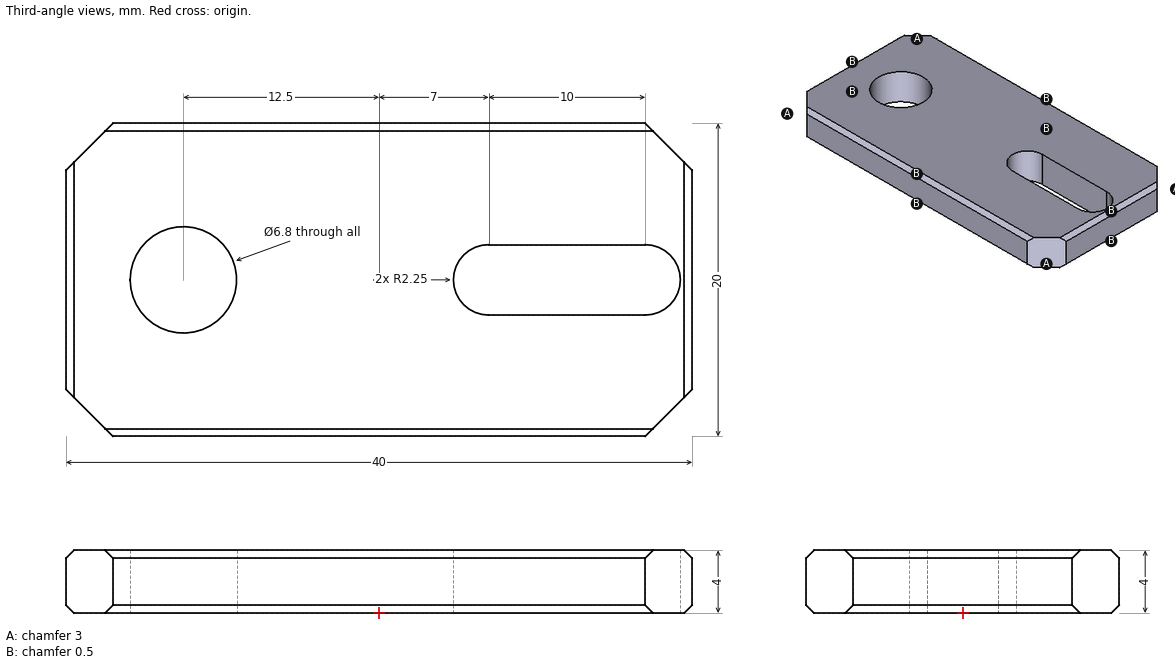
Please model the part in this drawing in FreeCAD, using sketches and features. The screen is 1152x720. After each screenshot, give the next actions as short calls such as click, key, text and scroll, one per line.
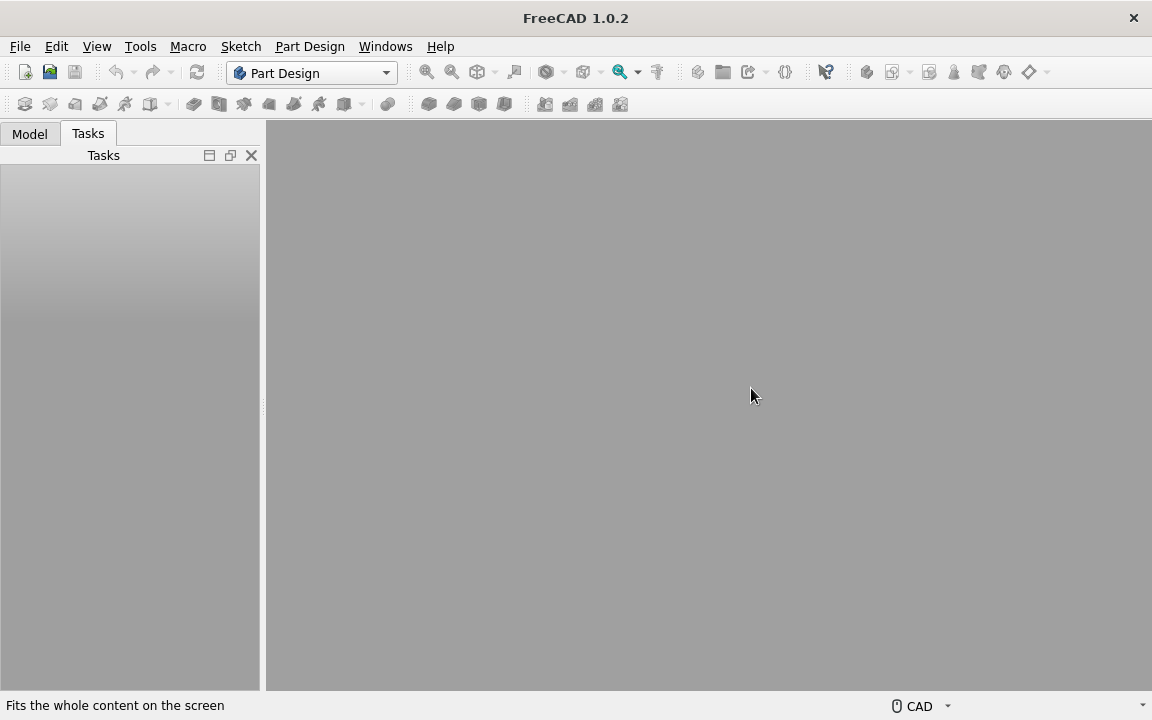
click(25, 72)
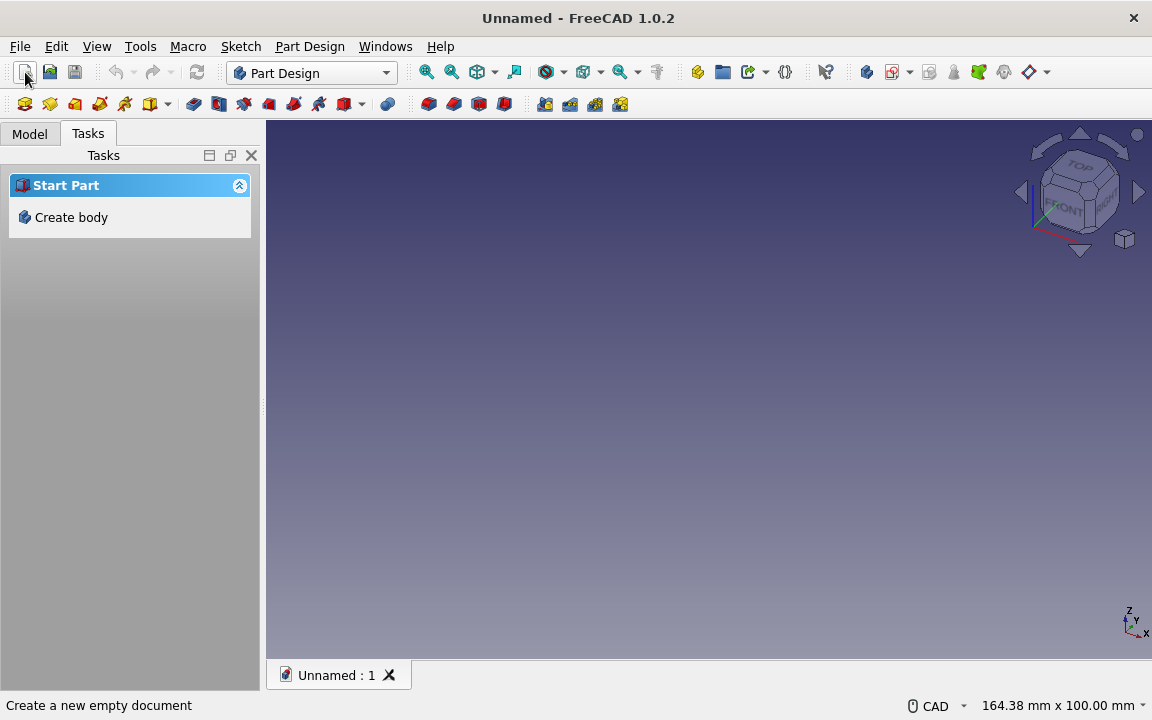
click(892, 72)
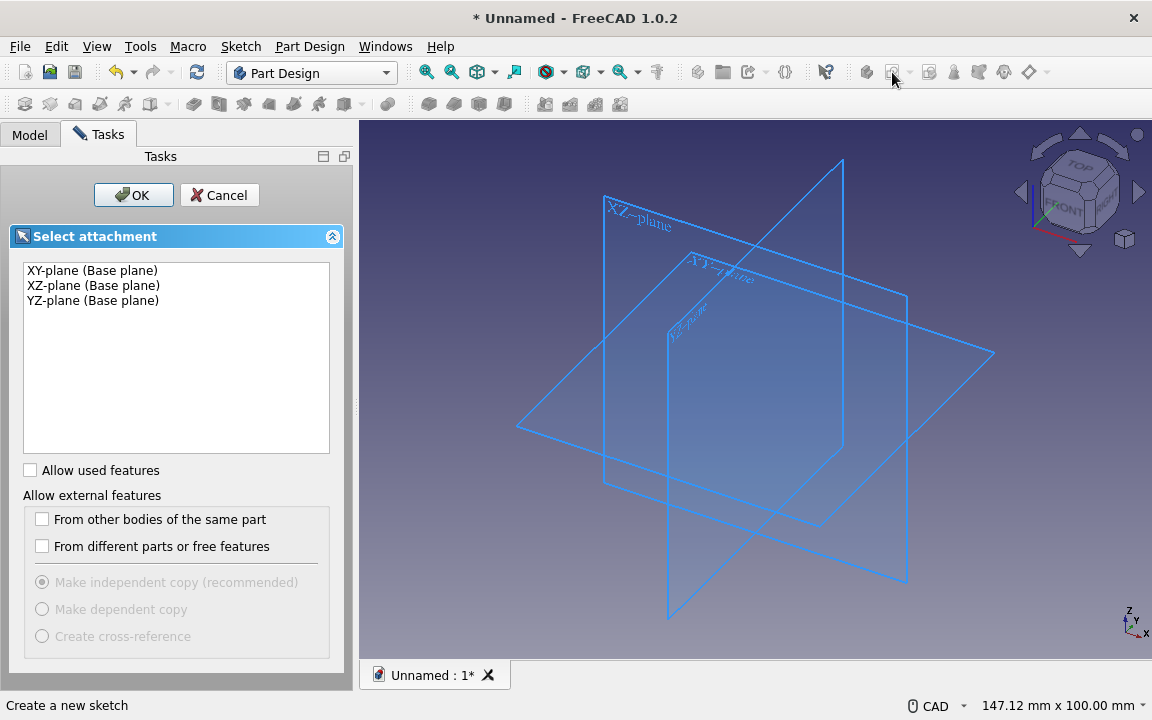
click(84, 270)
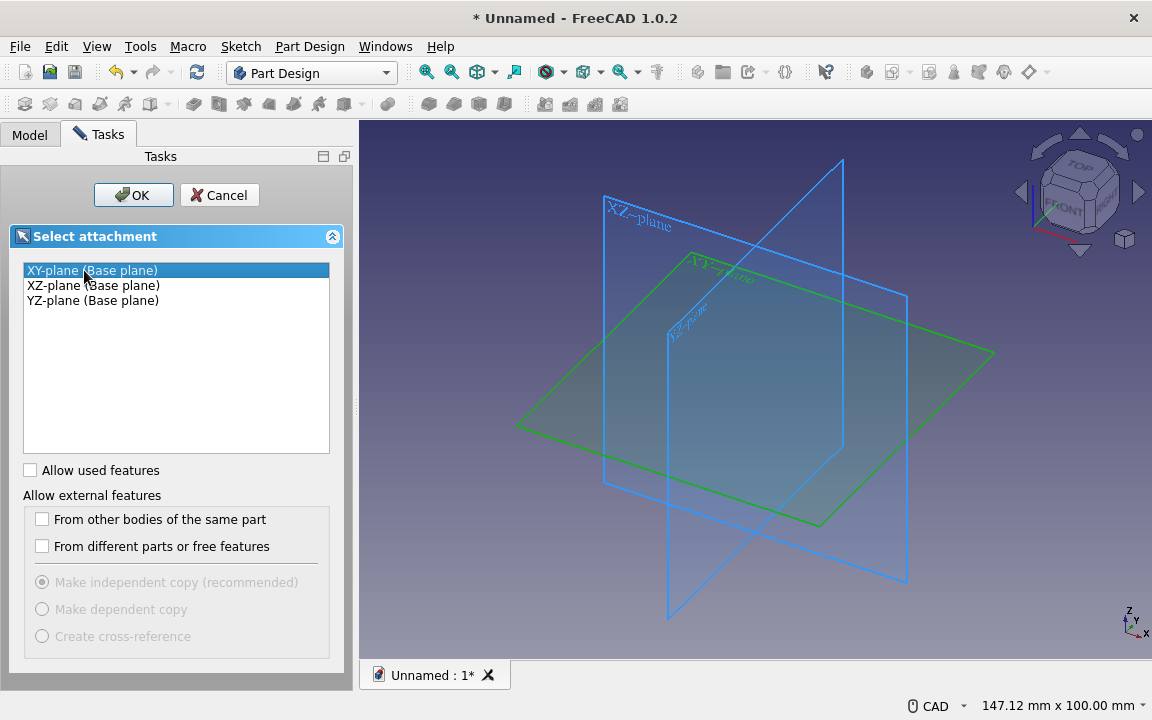
click(134, 195)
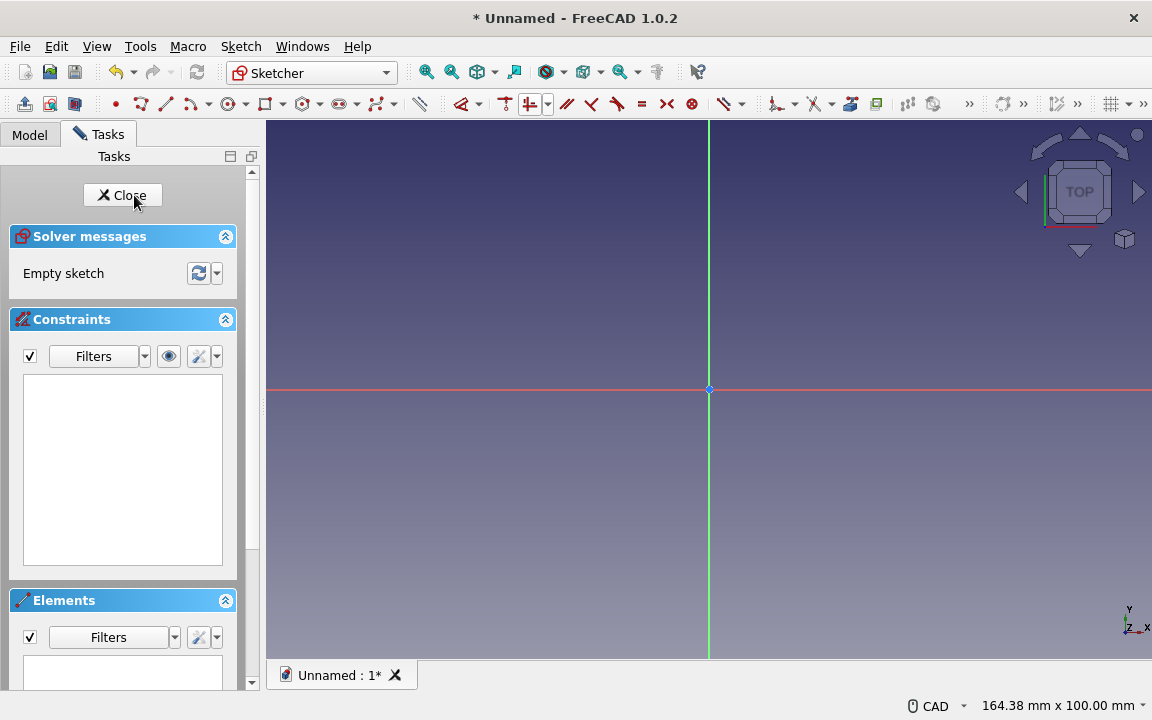
scroll(765, 390, up, 4)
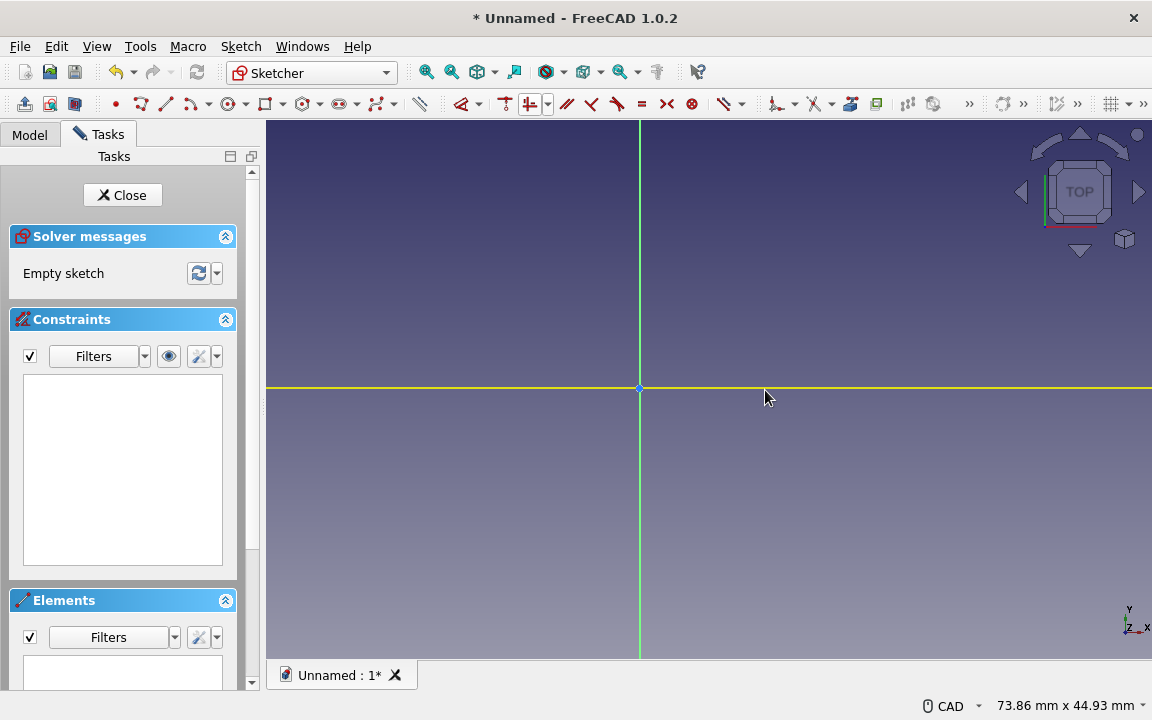
click(282, 104)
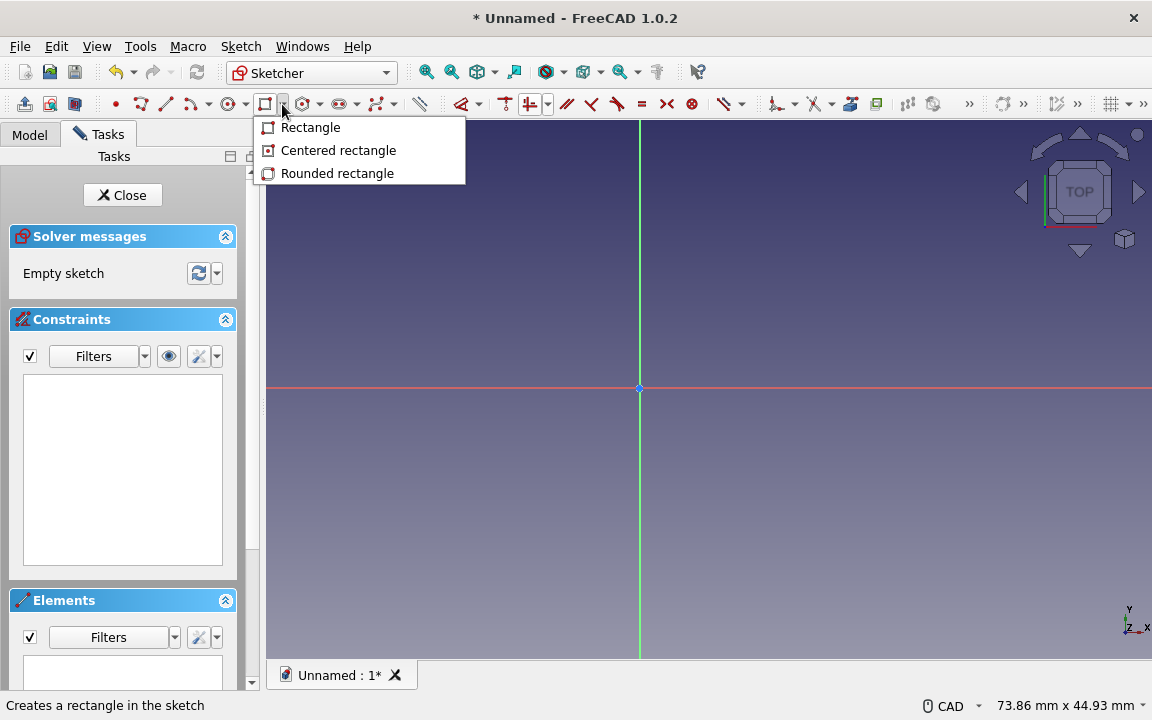
click(360, 150)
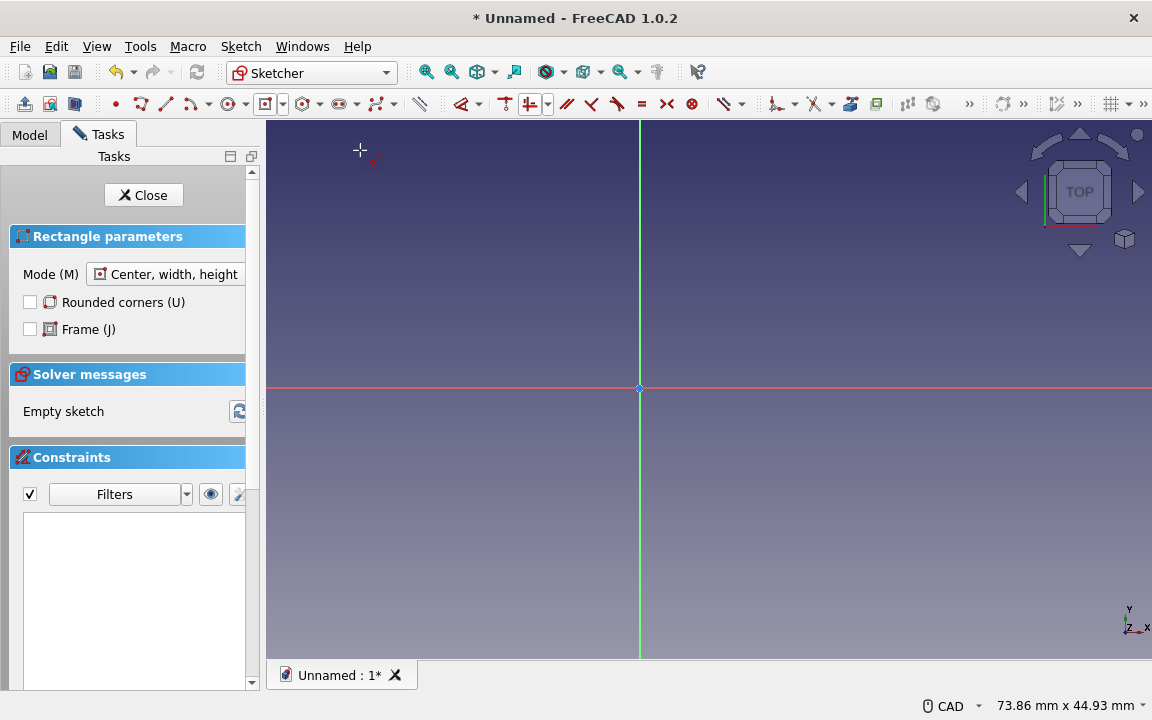
click(640, 388)
click(880, 268)
key(Escape)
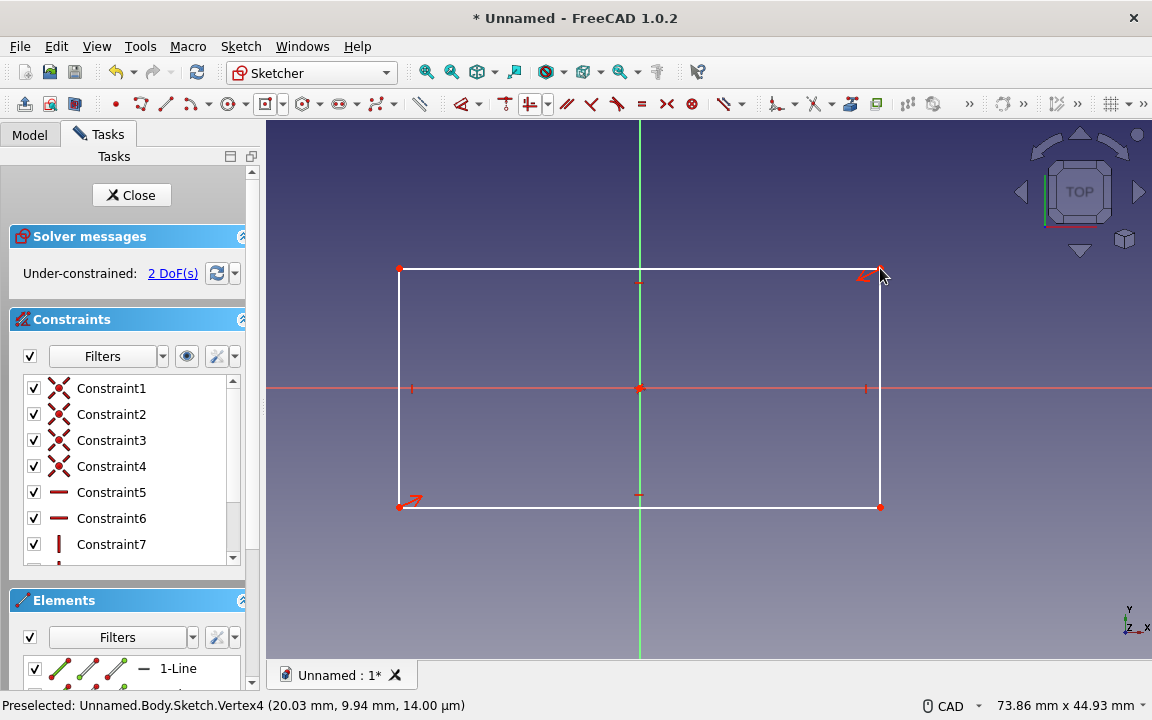
click(460, 104)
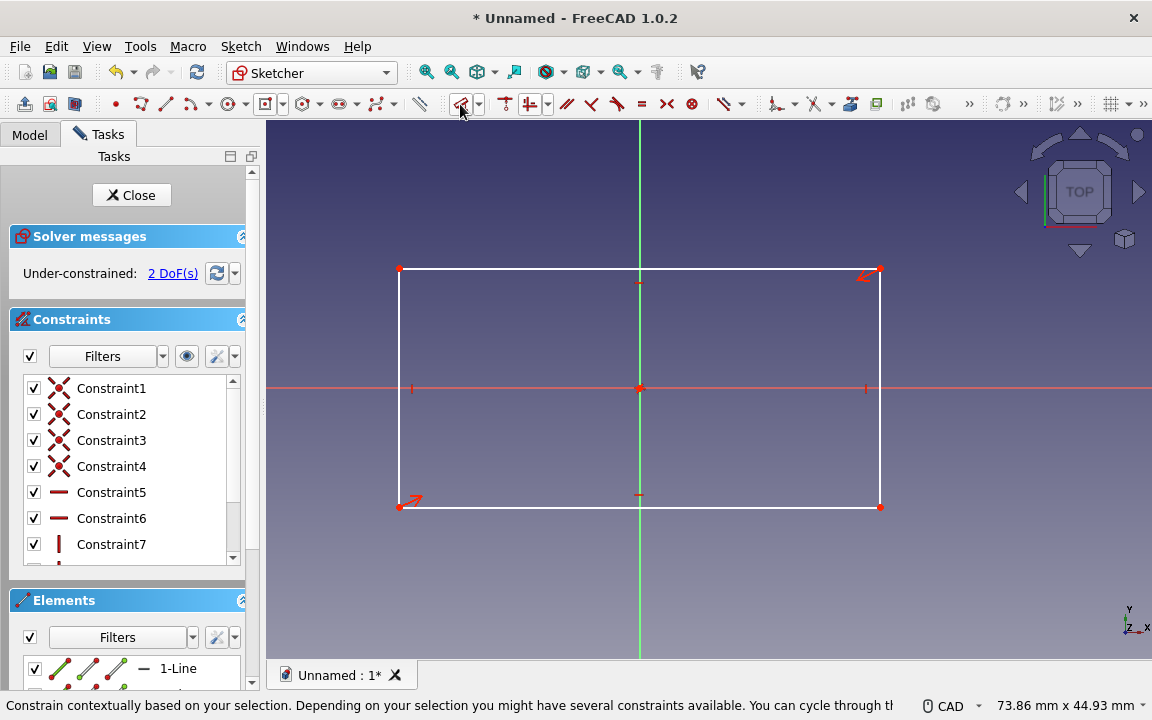
click(544, 508)
click(529, 542)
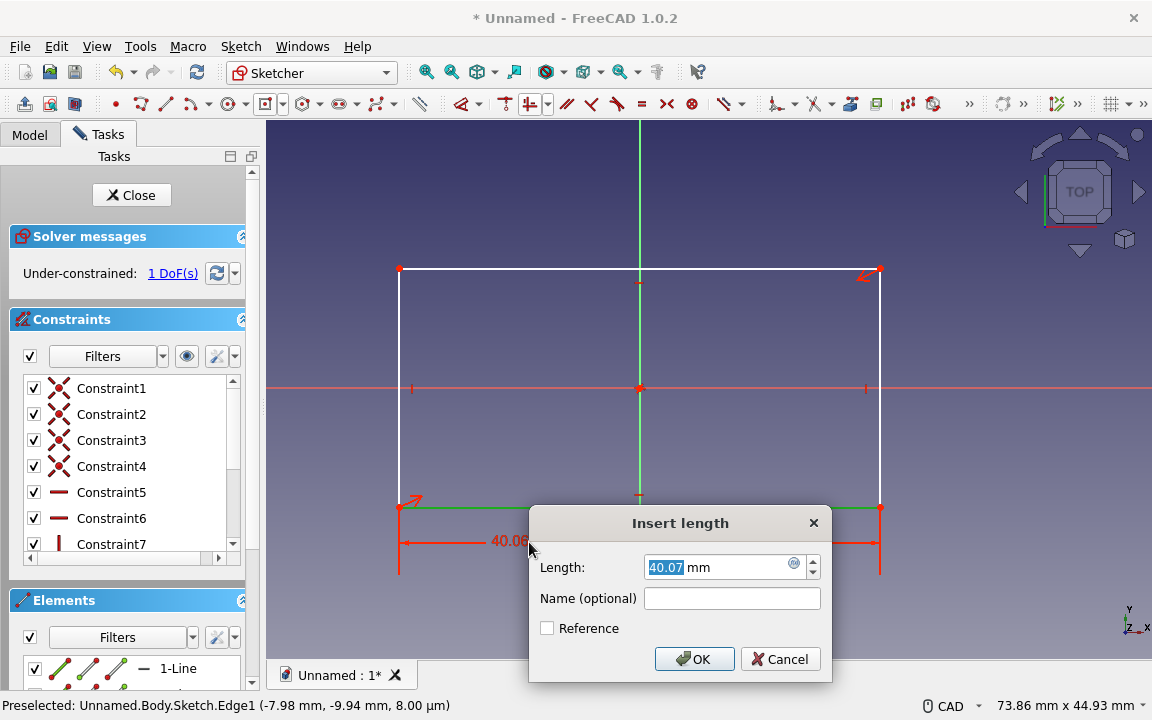
text(40)
key(Return)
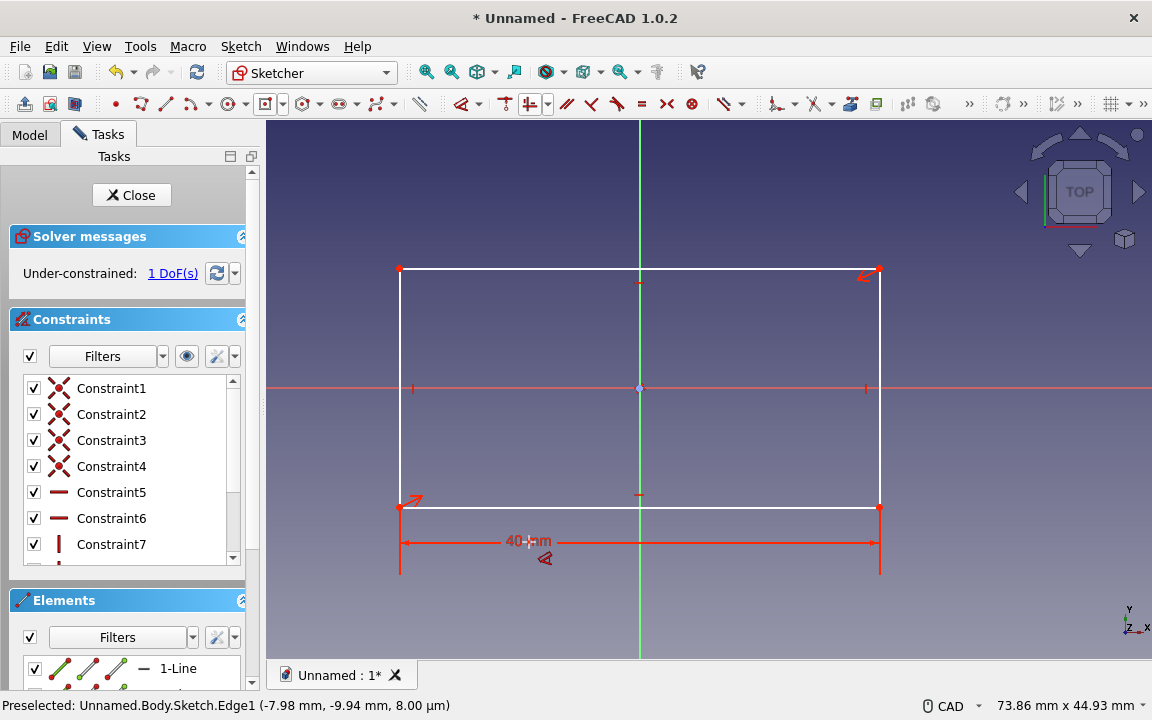
click(880, 436)
click(914, 333)